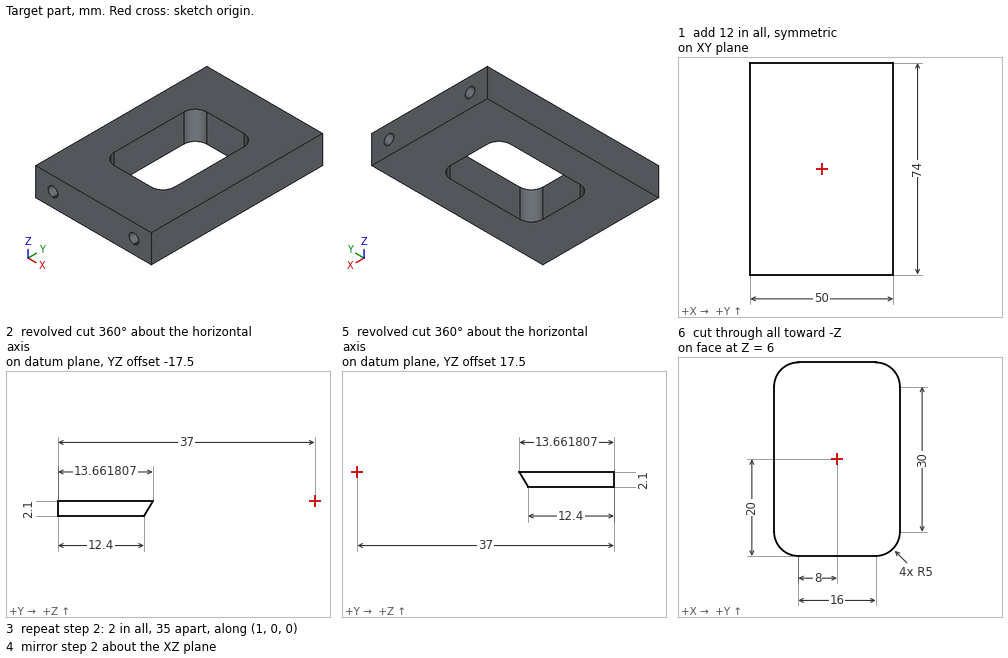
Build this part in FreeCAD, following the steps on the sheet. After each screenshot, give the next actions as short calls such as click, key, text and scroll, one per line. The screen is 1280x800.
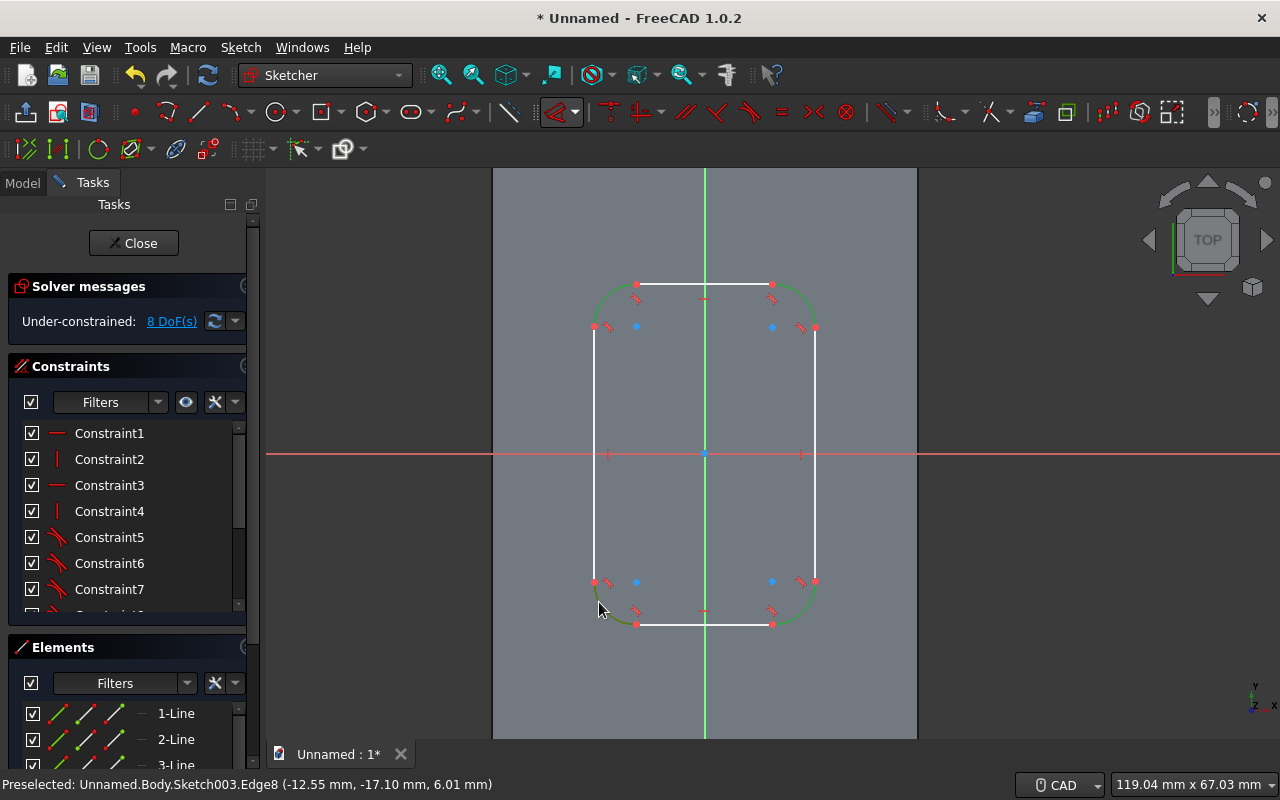
click(782, 112)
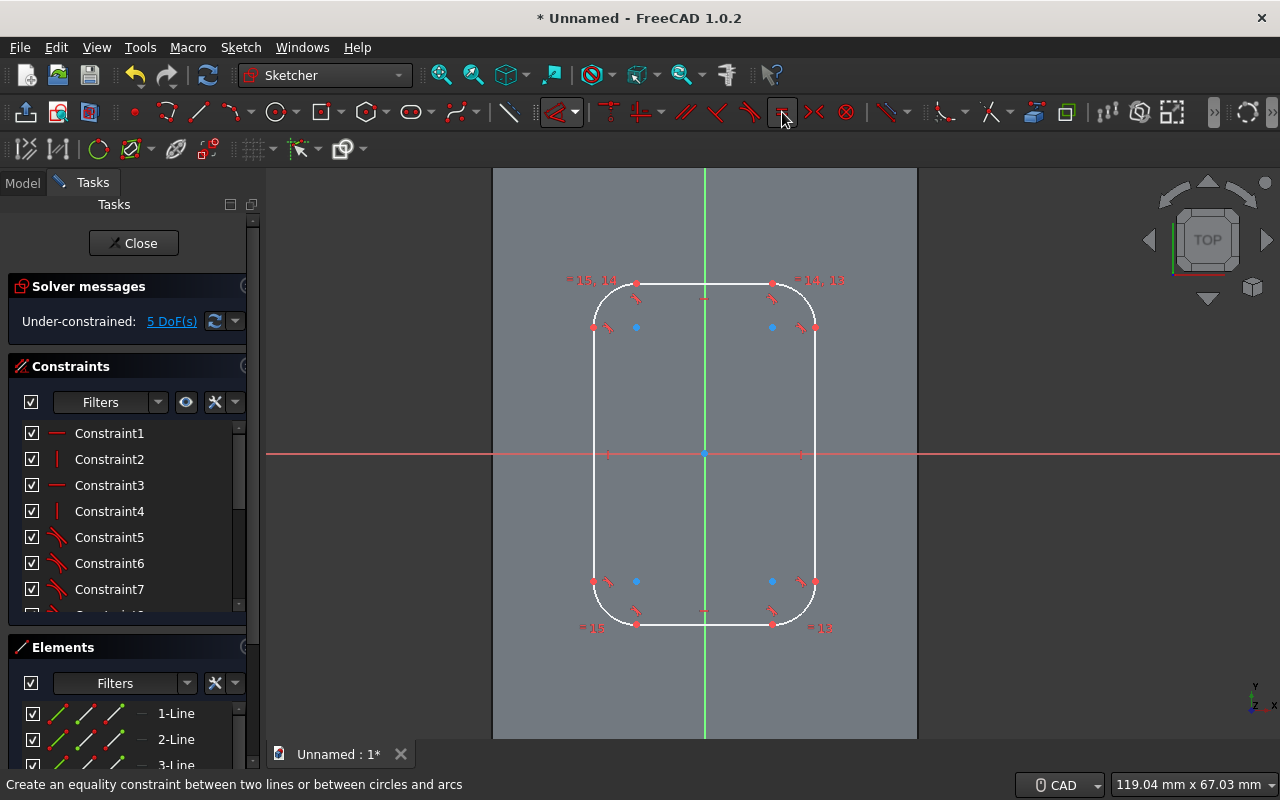
click(792, 620)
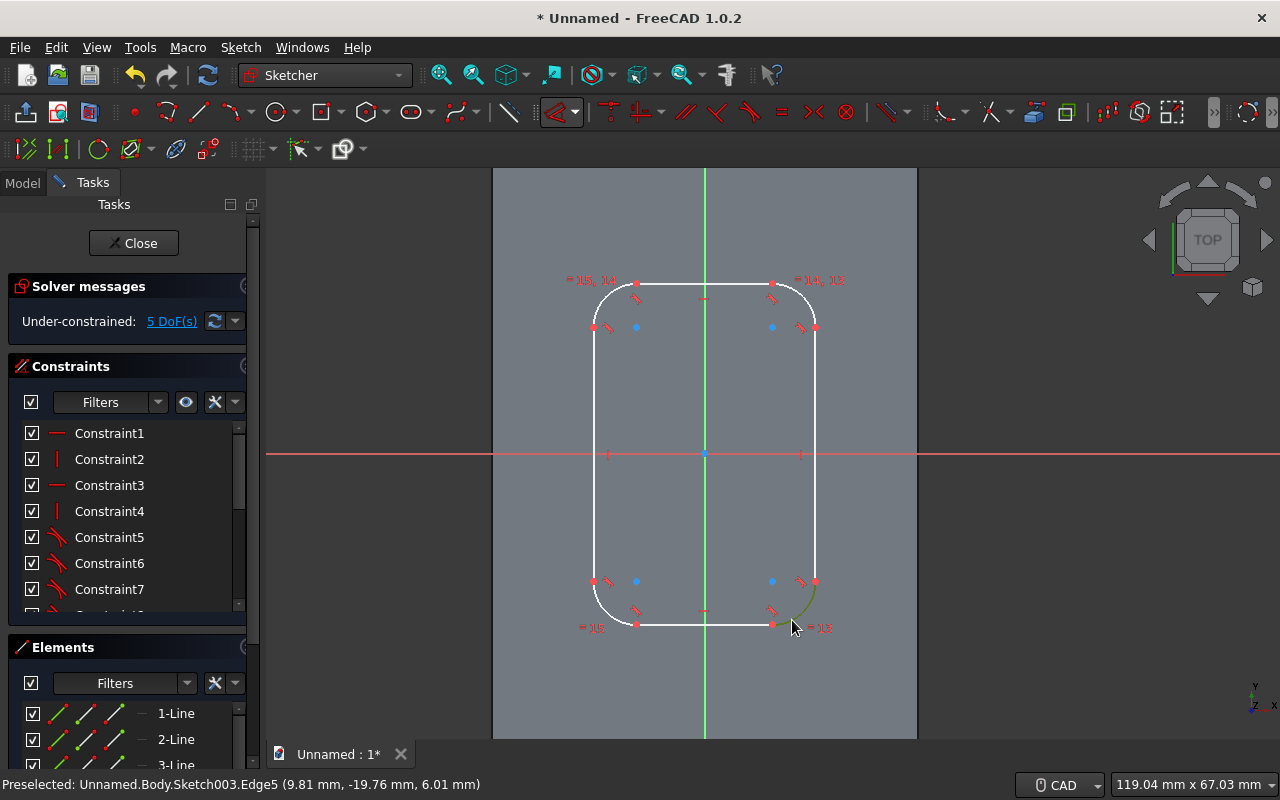
click(578, 112)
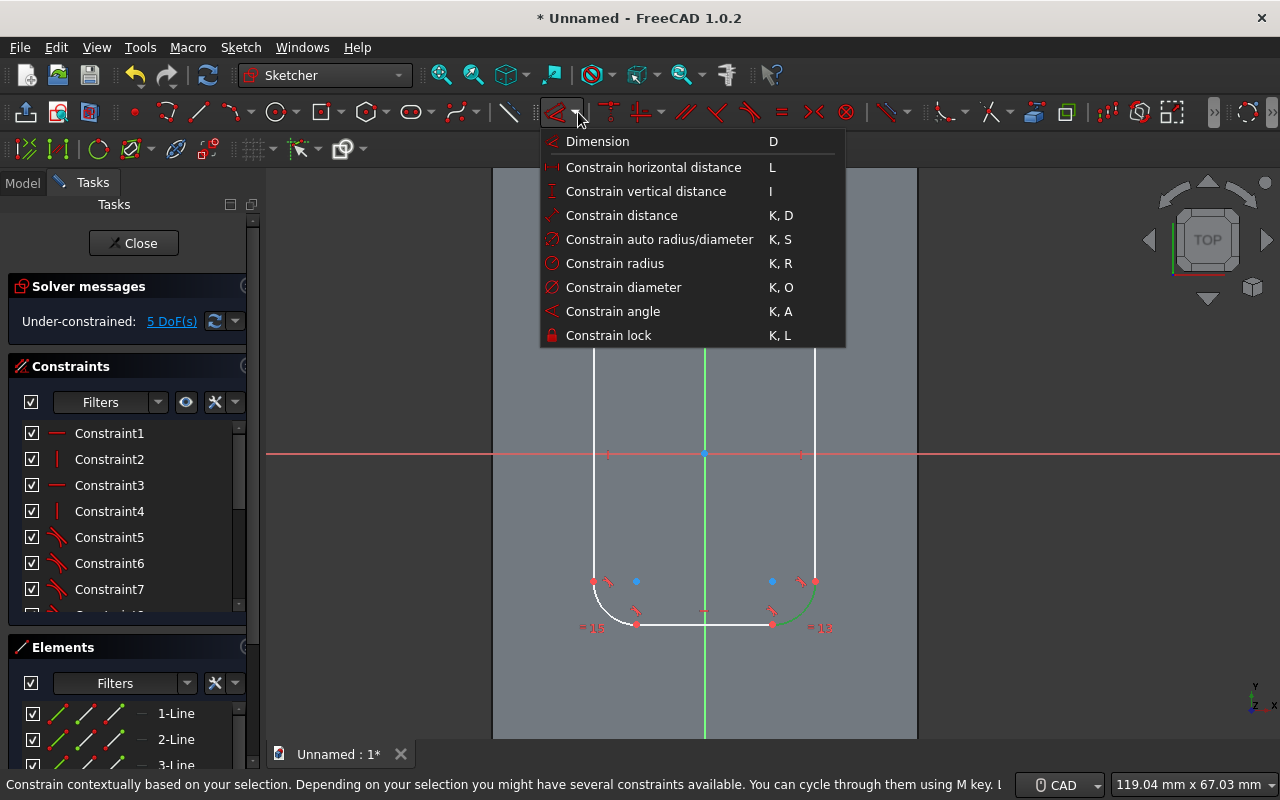
click(693, 263)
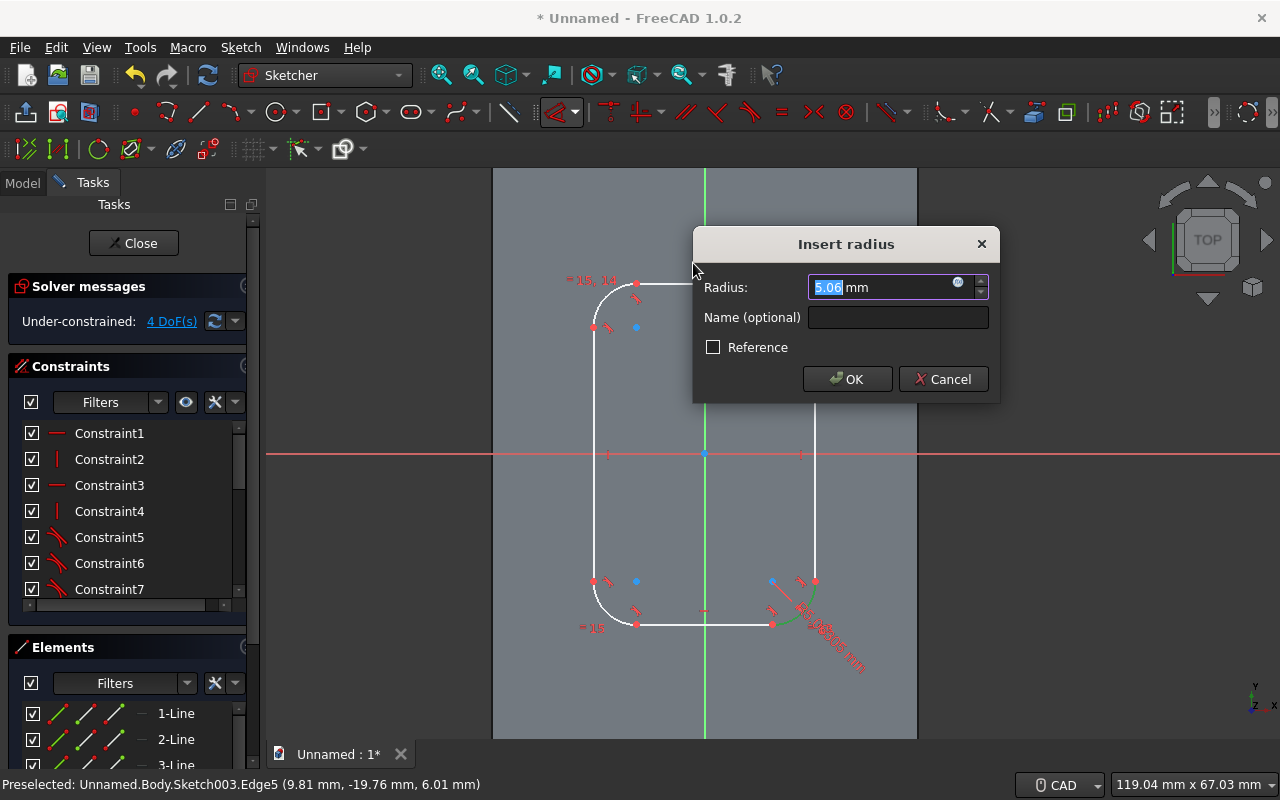
text(5)
key(Return)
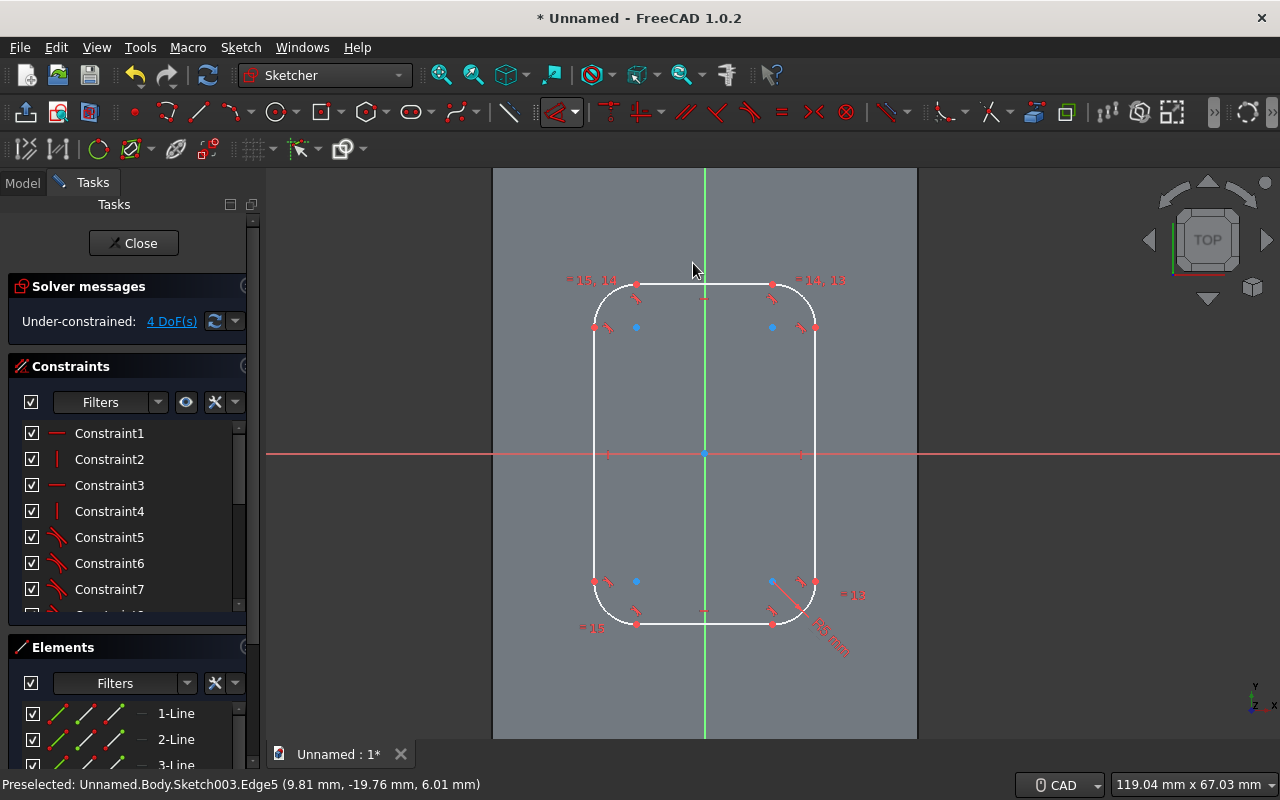
click(678, 624)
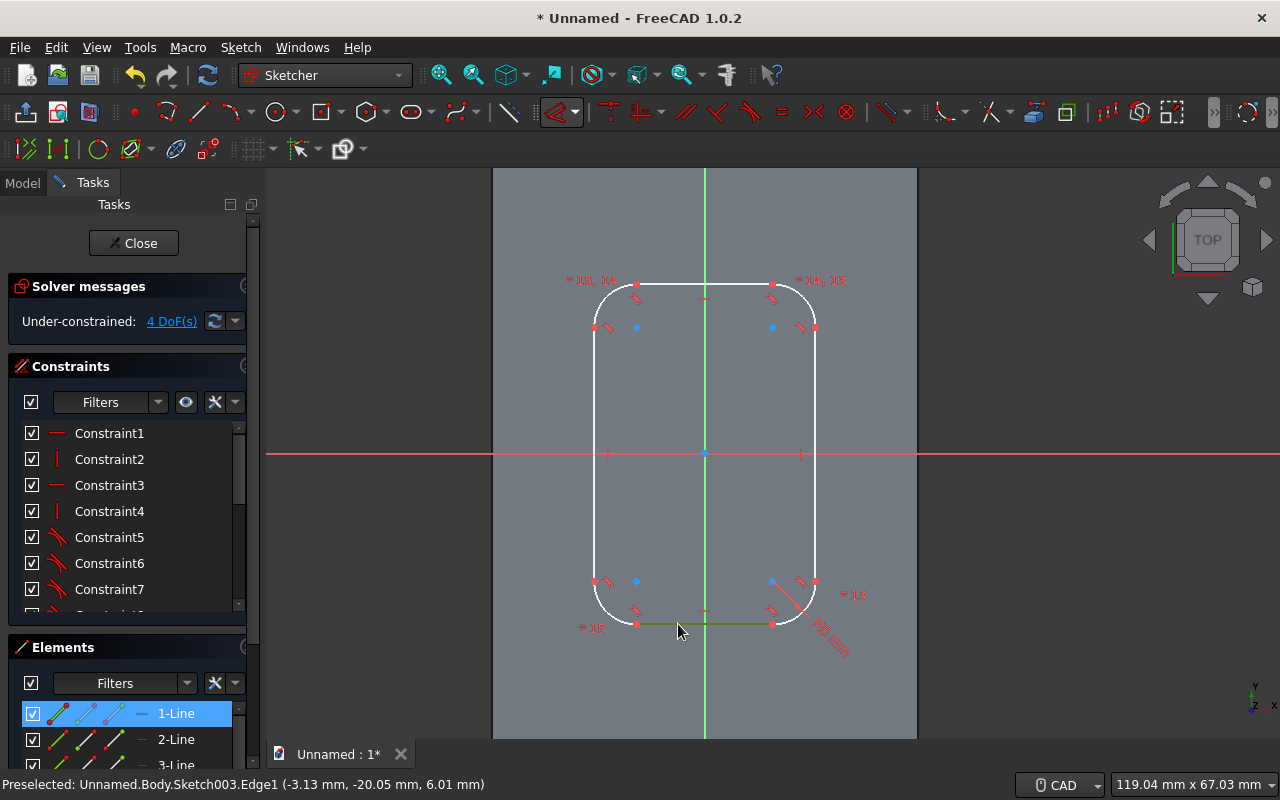
key(l)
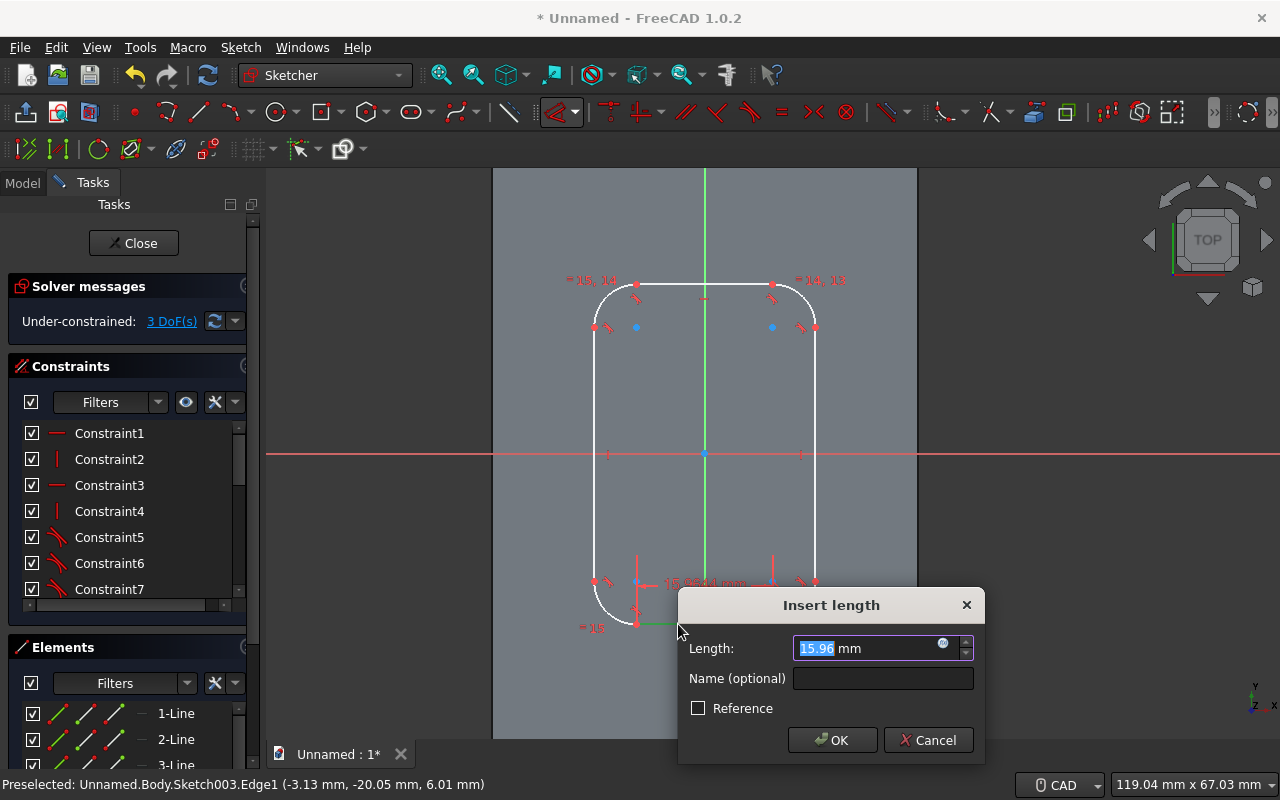
text(16)
key(Return)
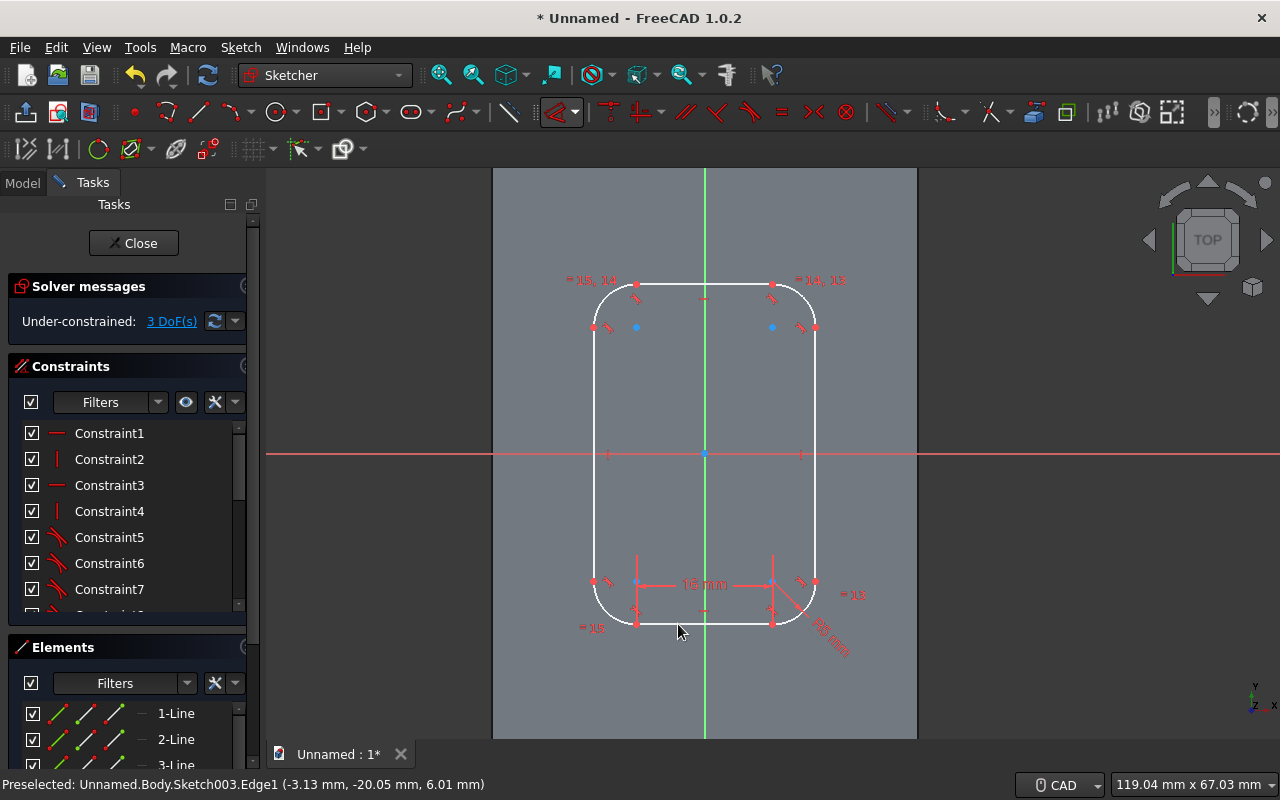
click(815, 505)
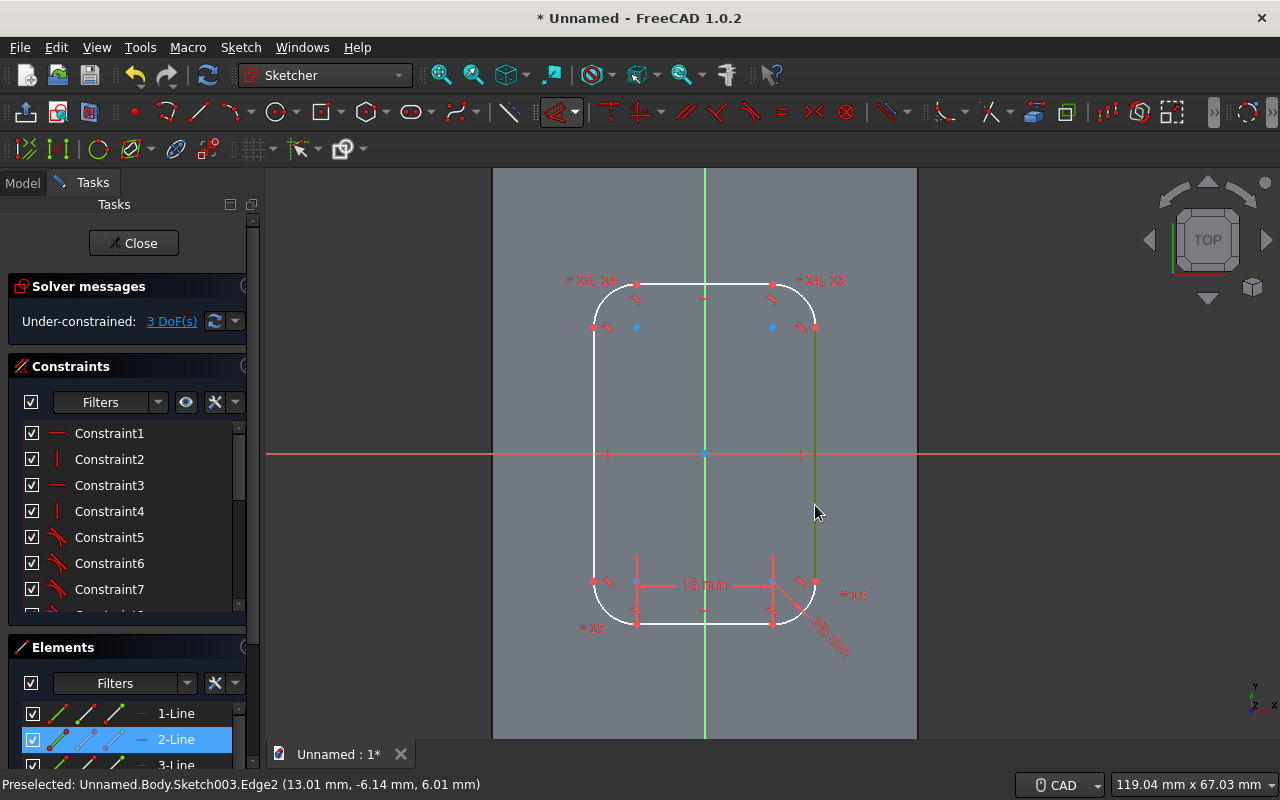
key(i)